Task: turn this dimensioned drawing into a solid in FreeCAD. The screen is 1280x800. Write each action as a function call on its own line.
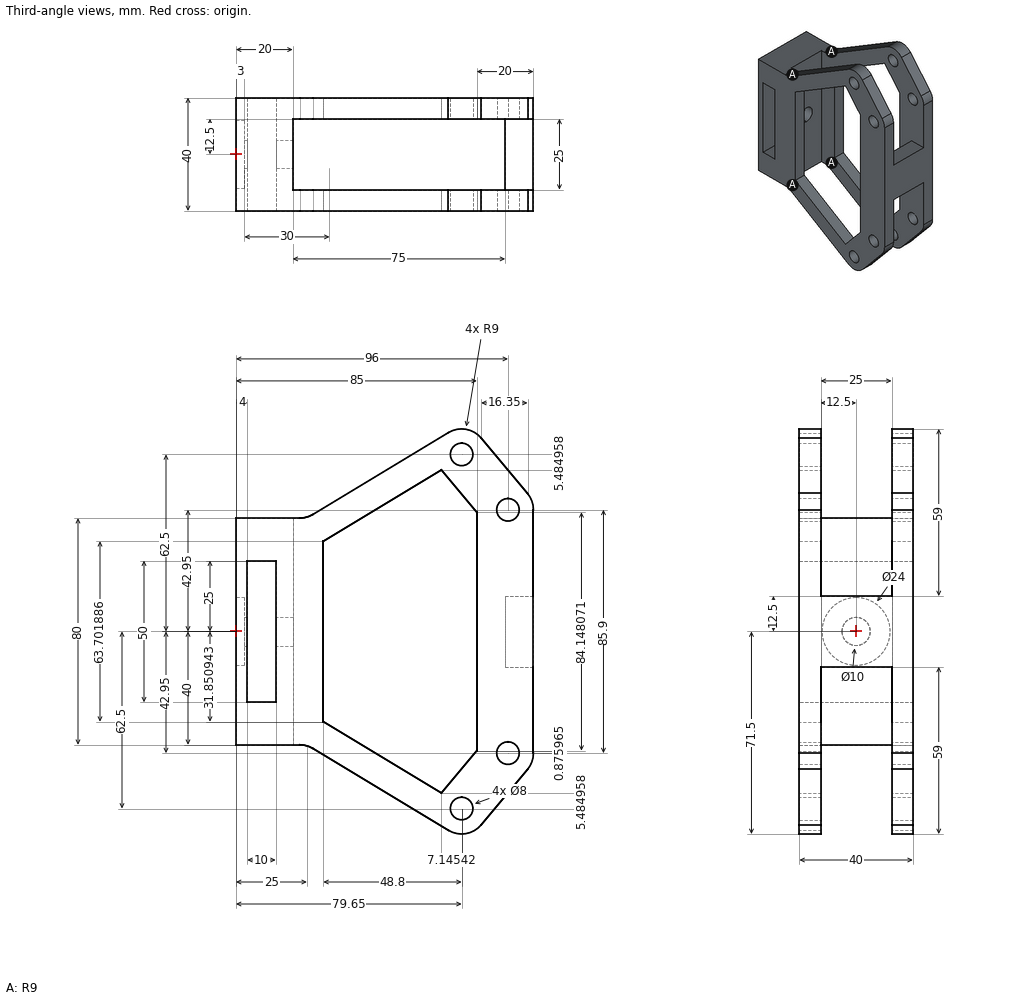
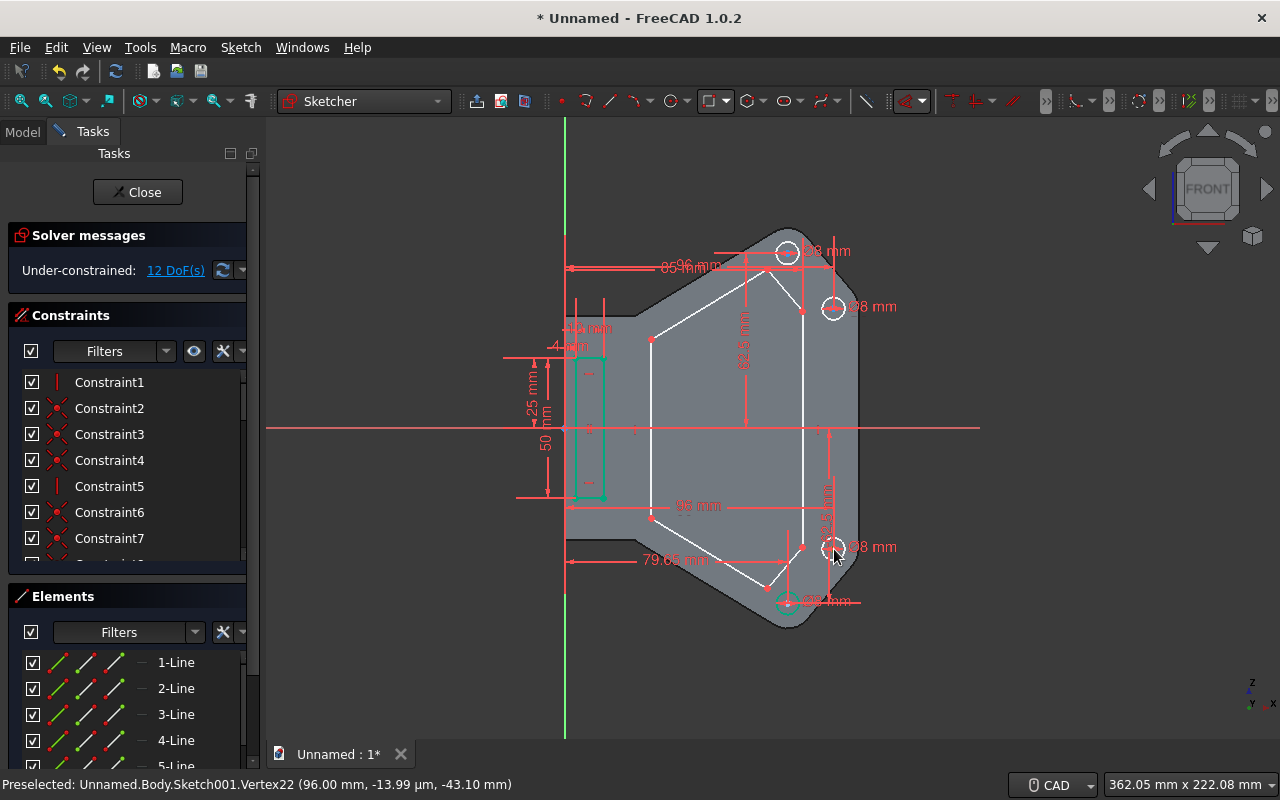
click(924, 102)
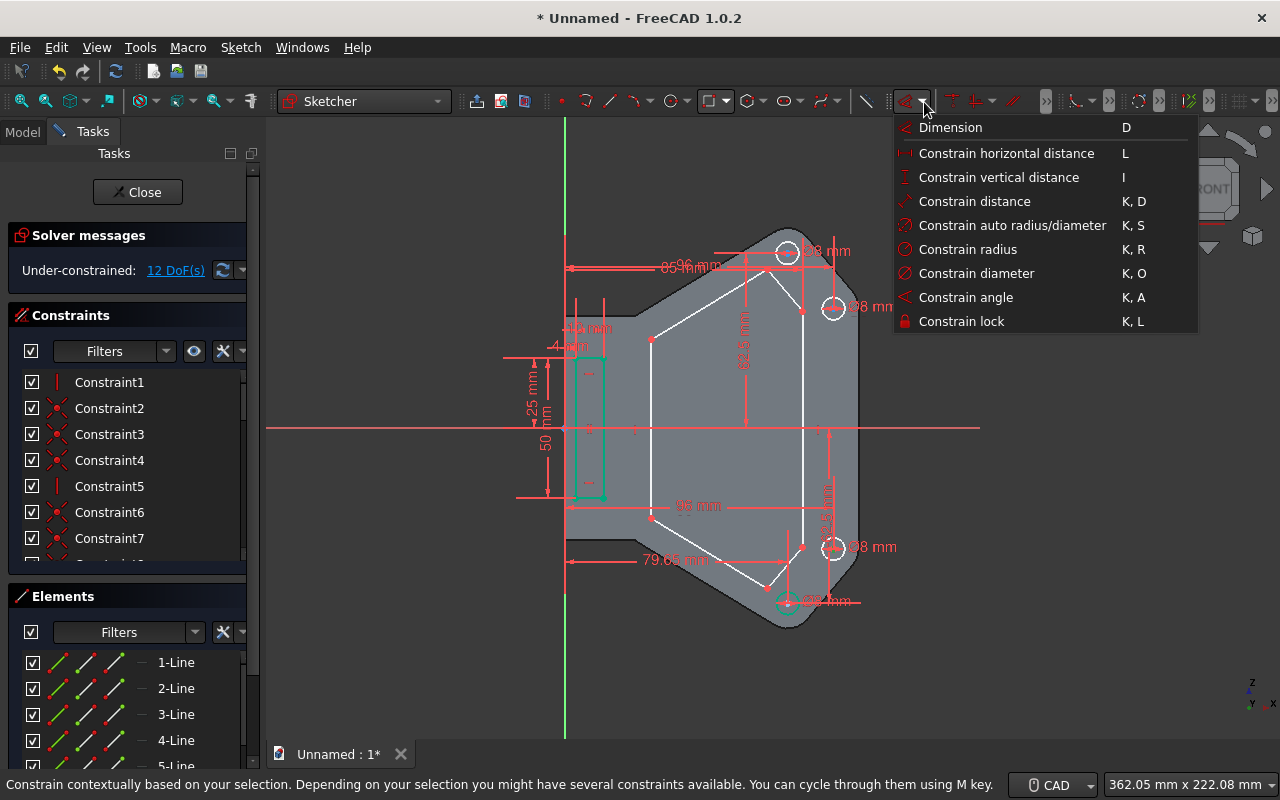
click(1046, 177)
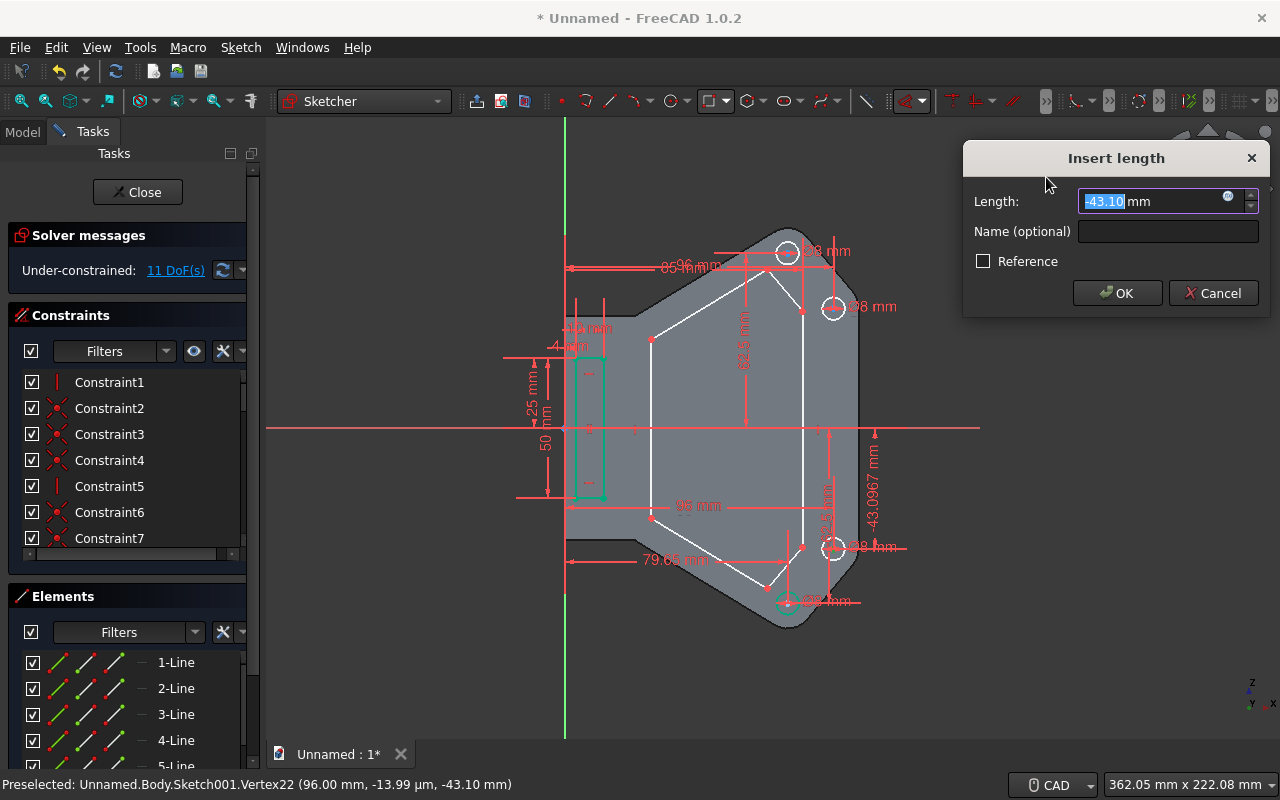
text(-42.95)
key(Return)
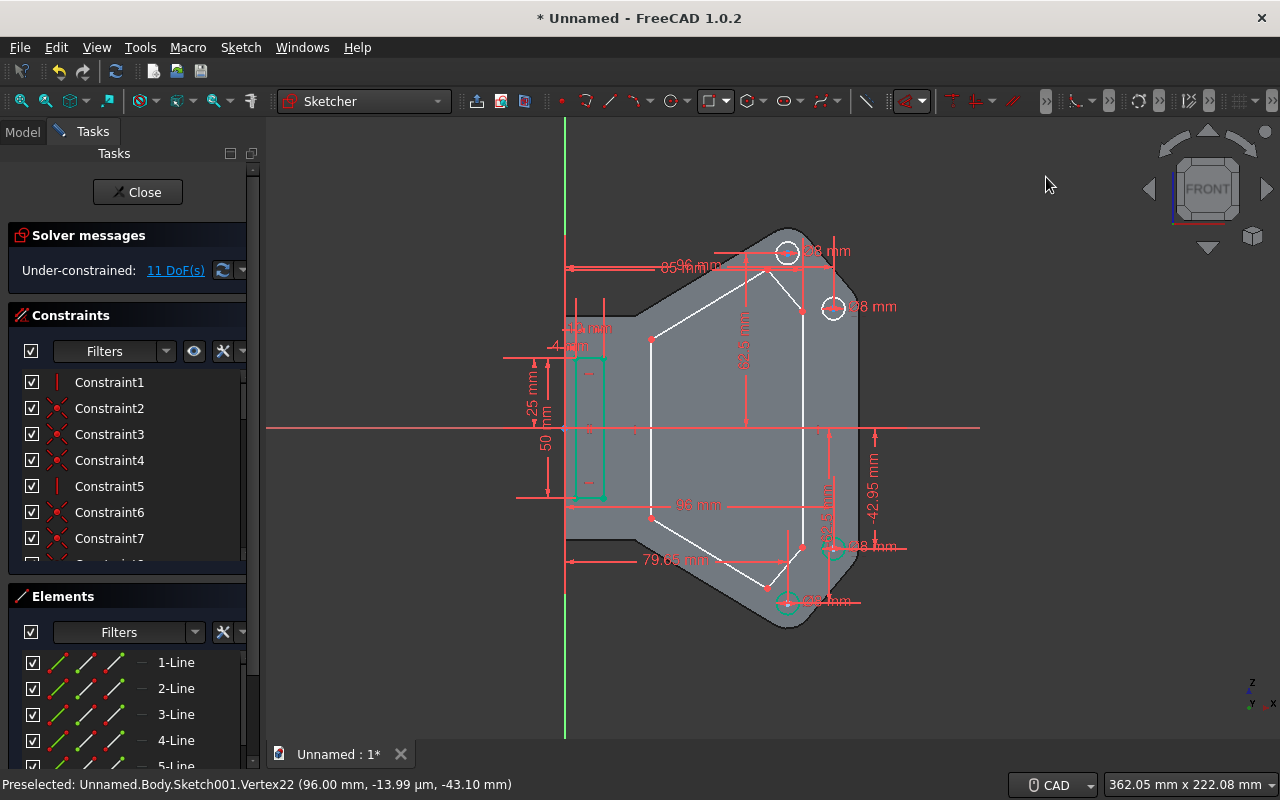
click(834, 309)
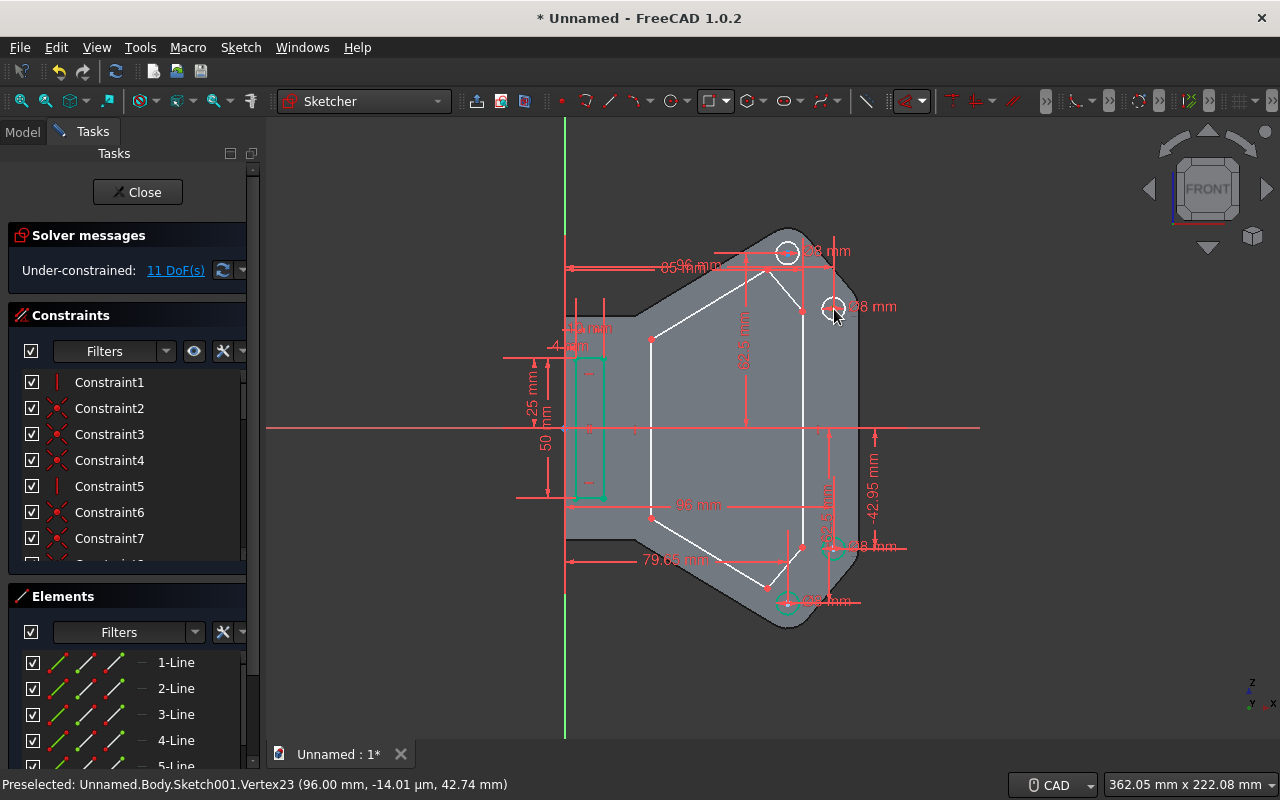
click(924, 102)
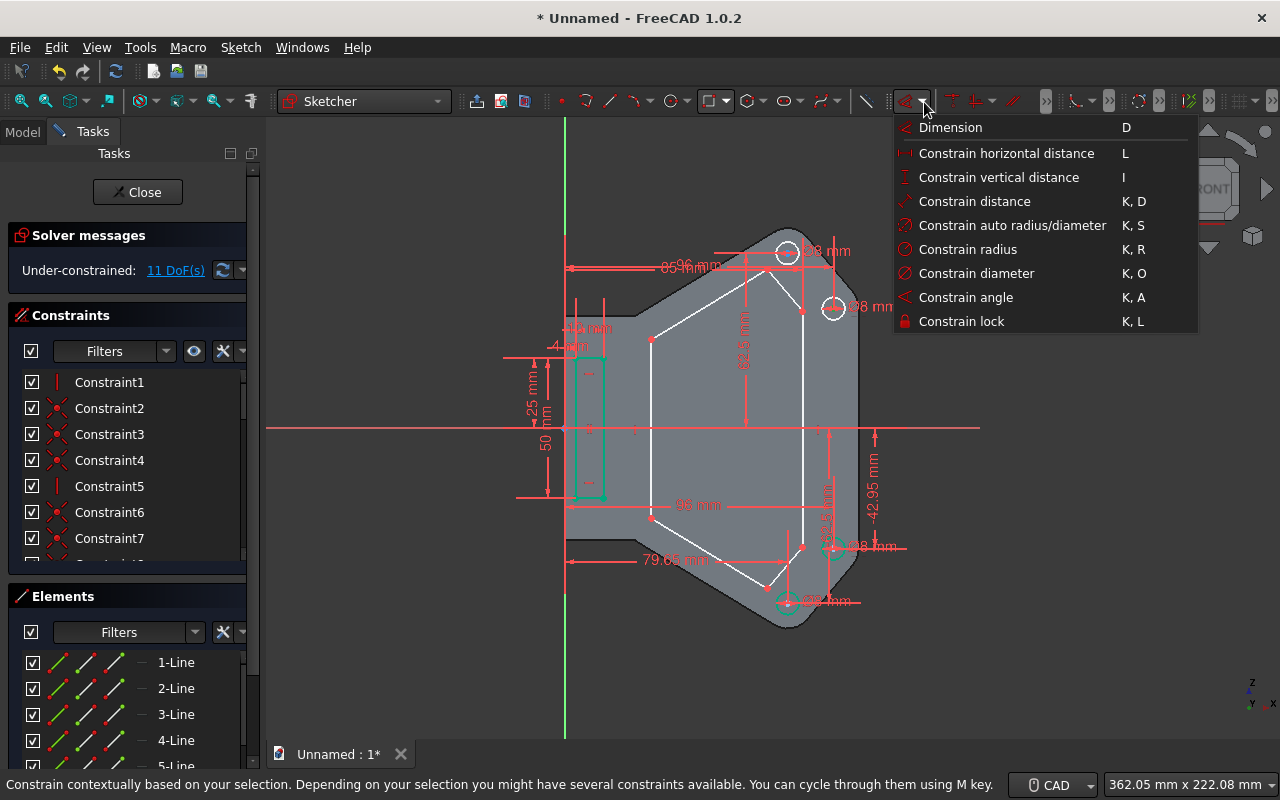
click(1046, 177)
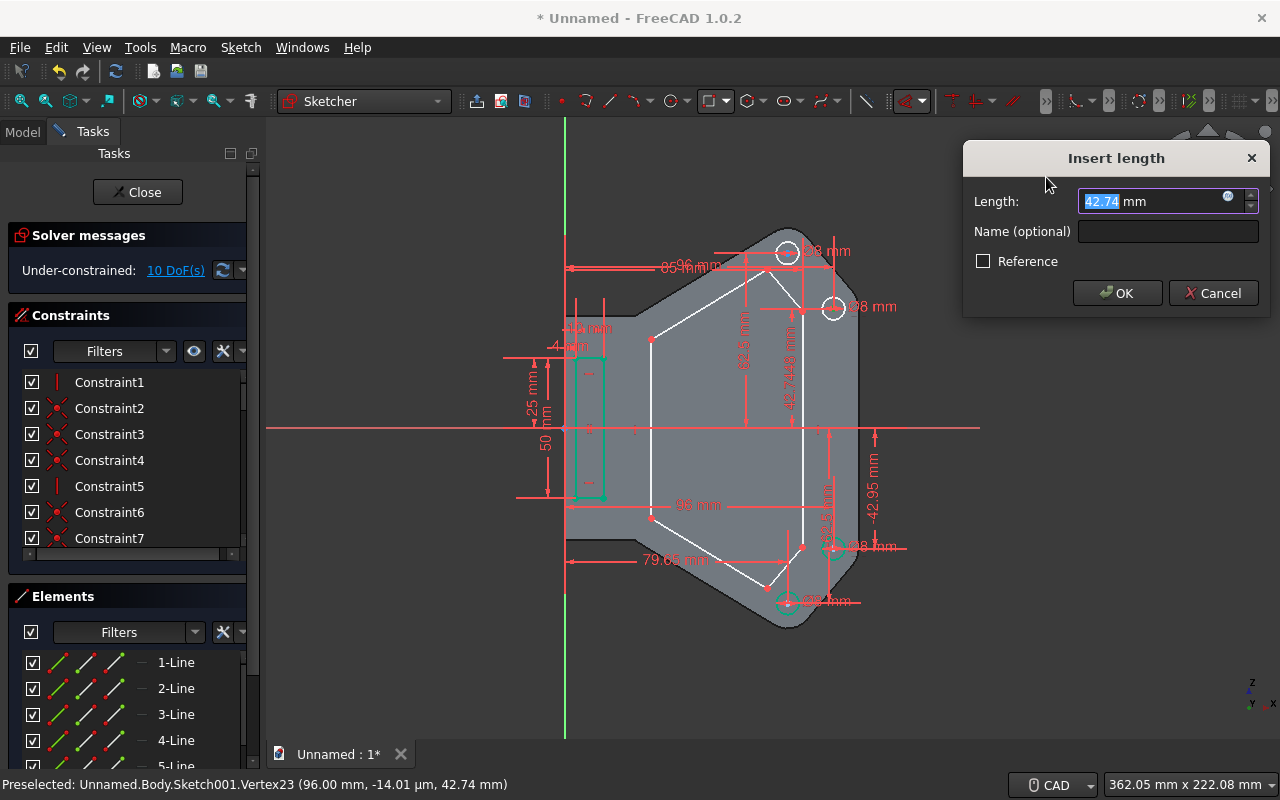
text(42.95)
key(Return)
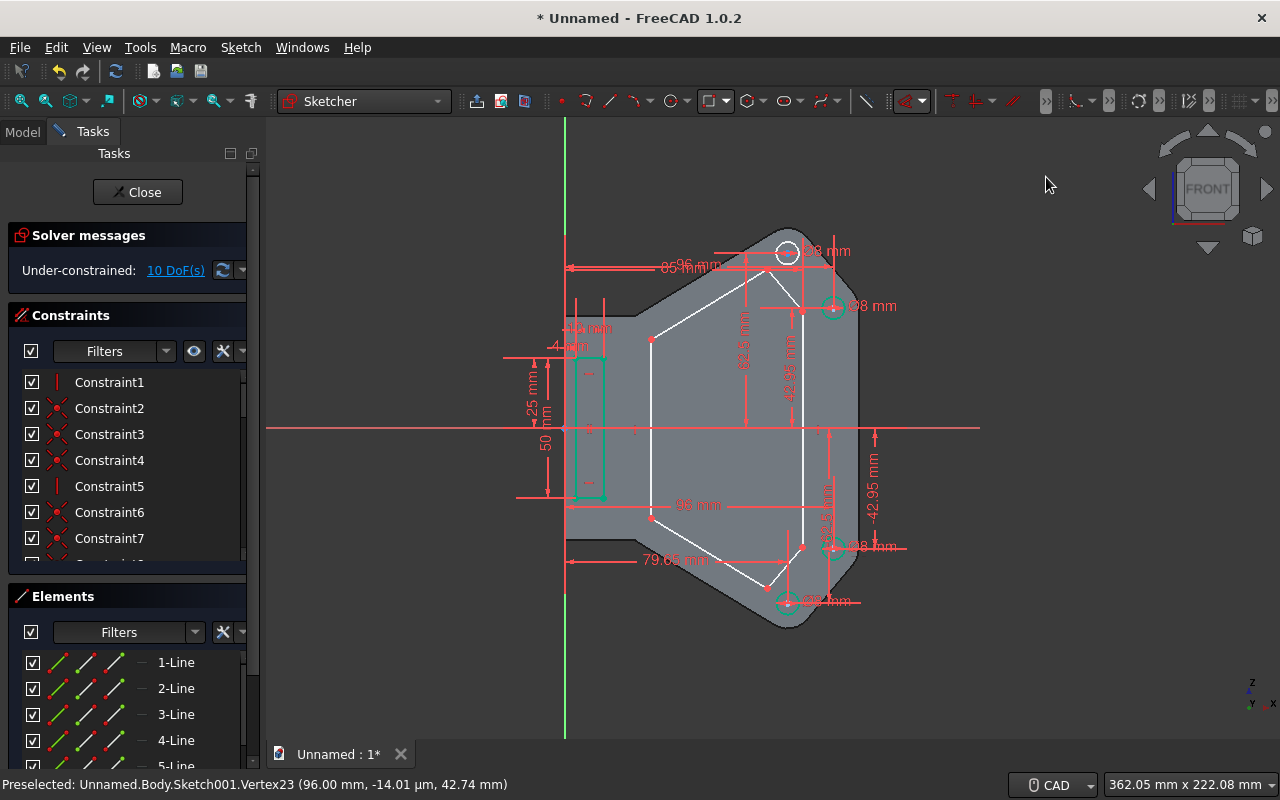
click(788, 253)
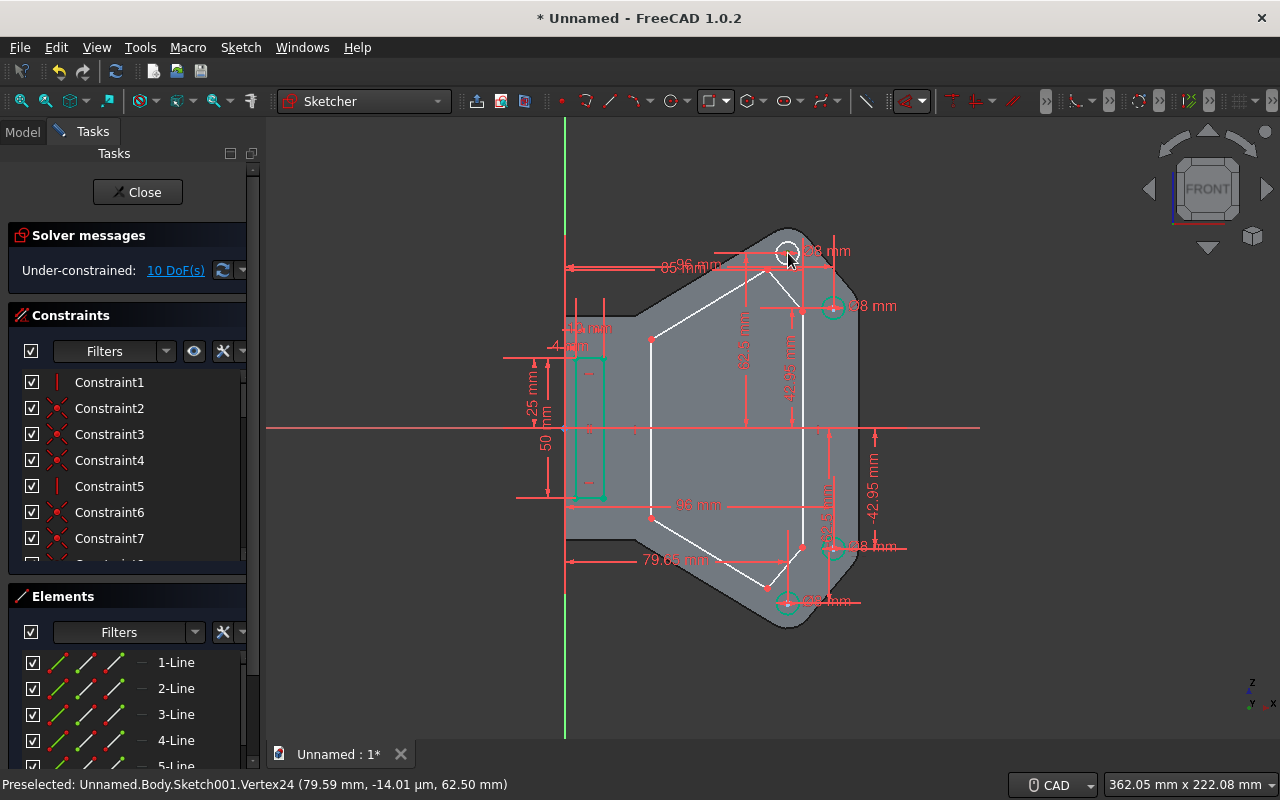
key(l)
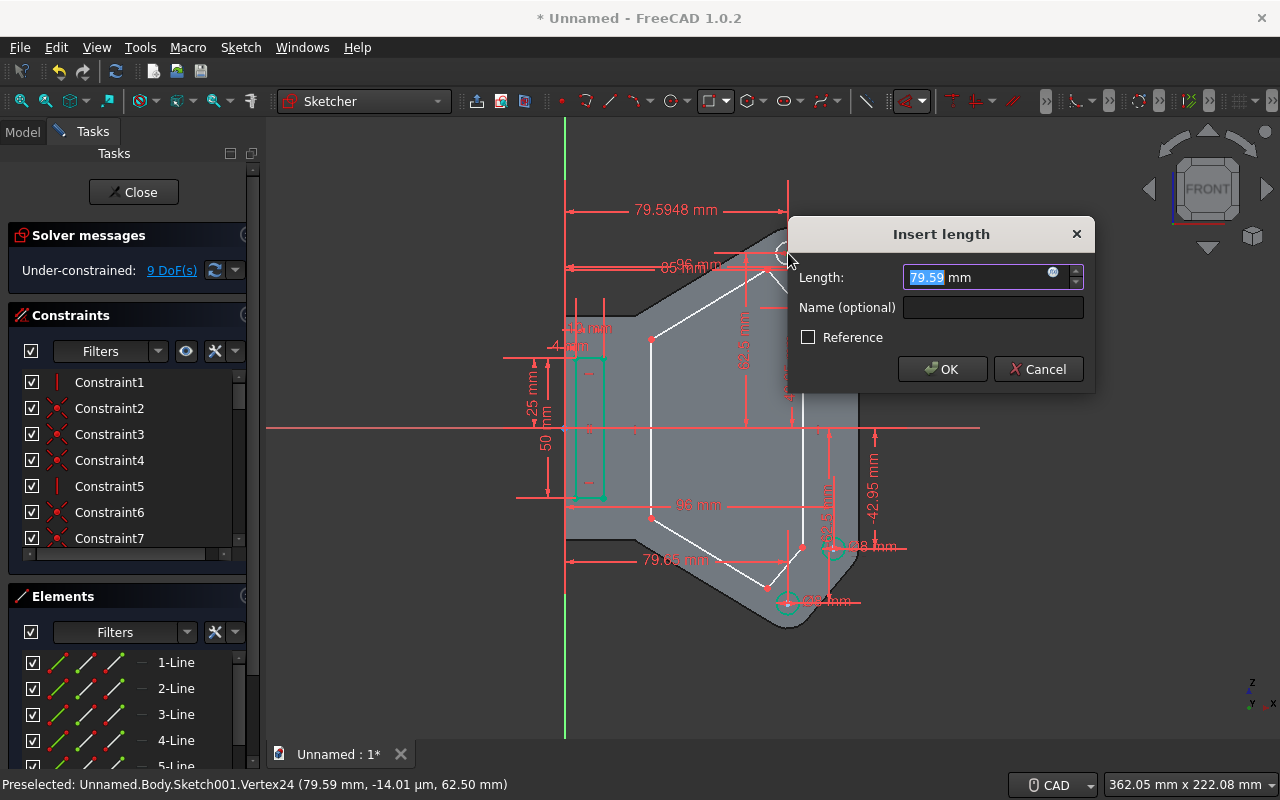
text(79.65)
key(Return)